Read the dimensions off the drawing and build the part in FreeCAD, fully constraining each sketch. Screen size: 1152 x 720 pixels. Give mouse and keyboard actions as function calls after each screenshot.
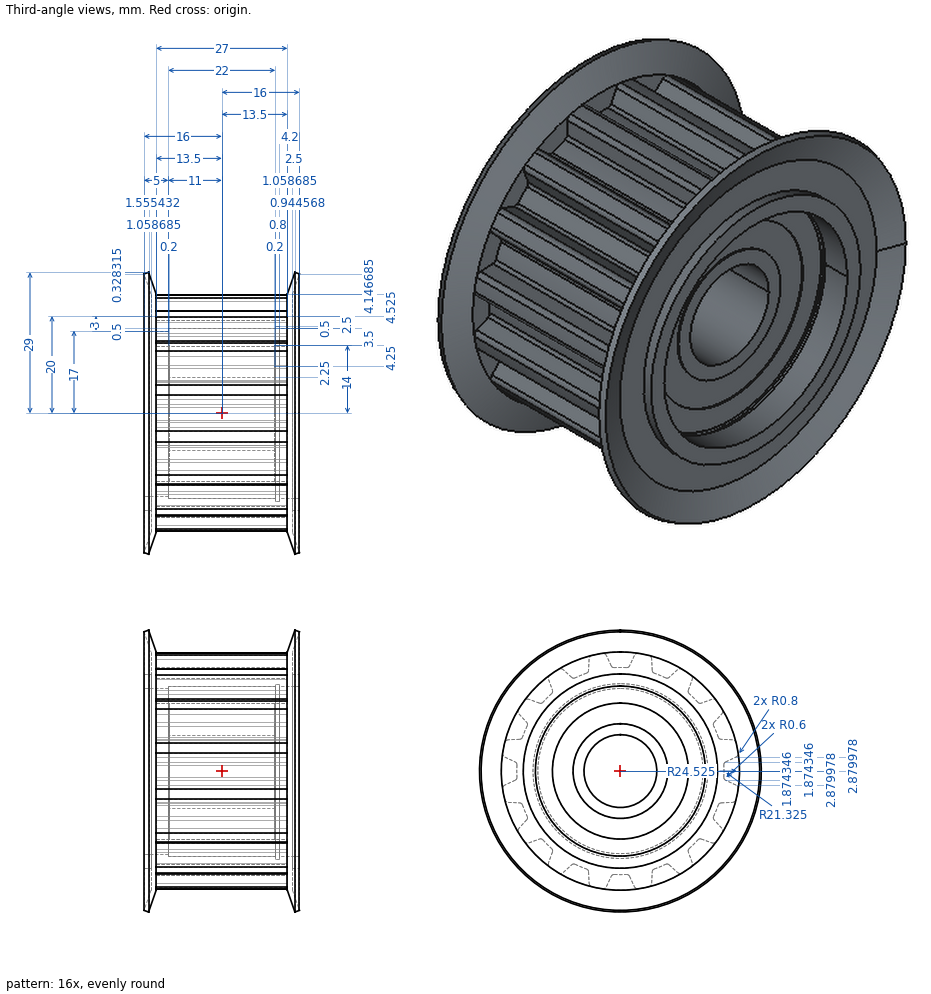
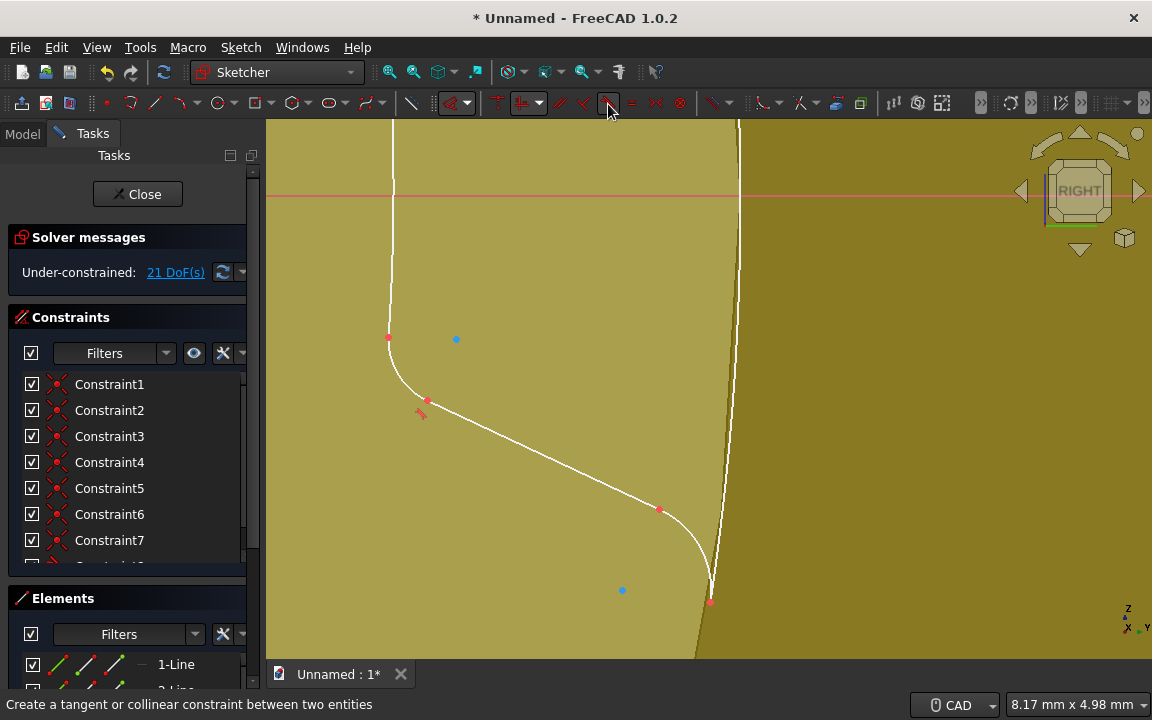
click(590, 477)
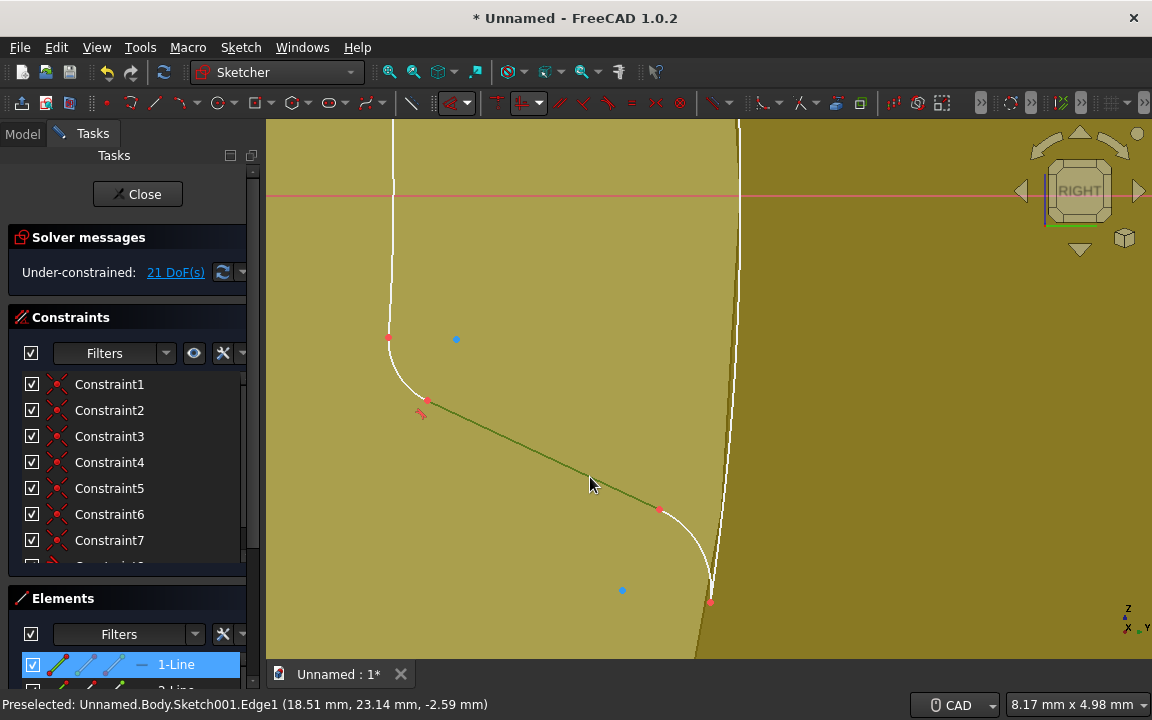
click(687, 530)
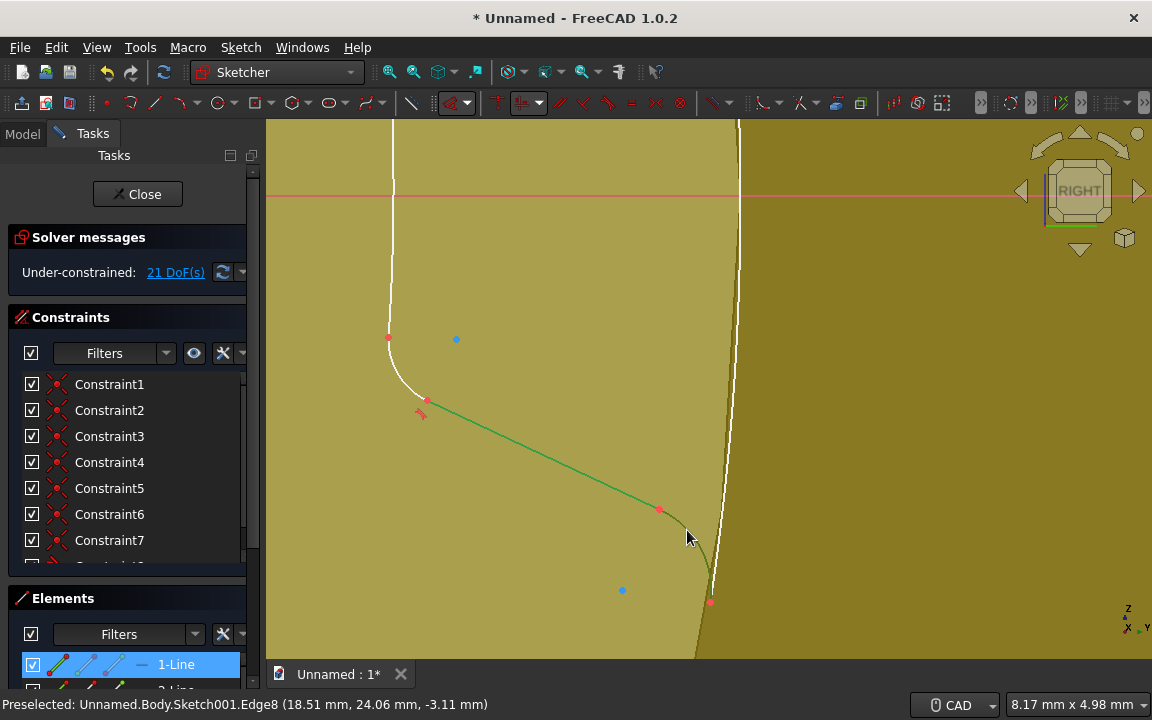
click(608, 104)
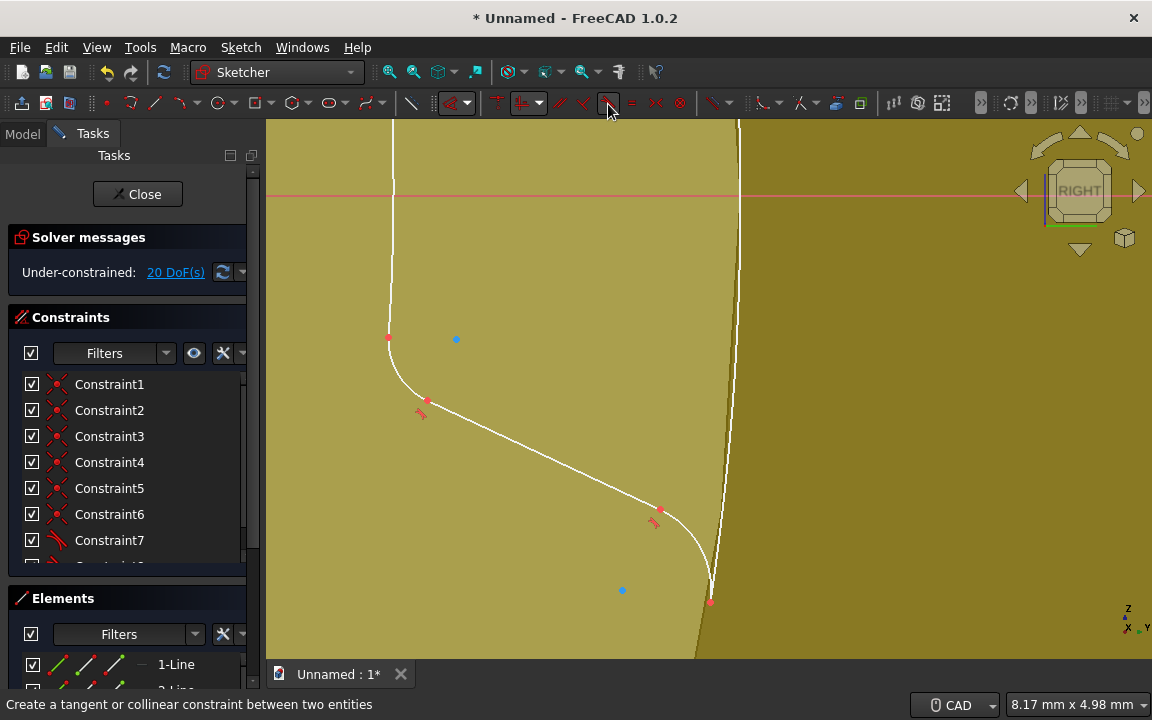
scroll(702, 546, down, 4)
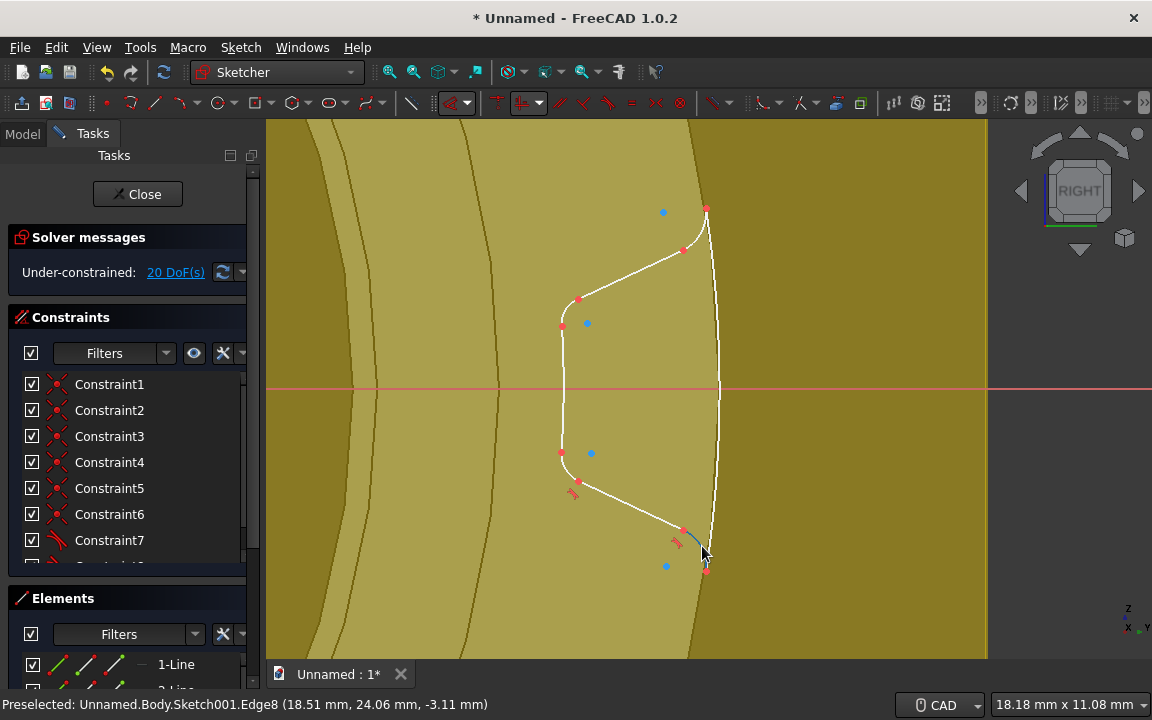
click(610, 285)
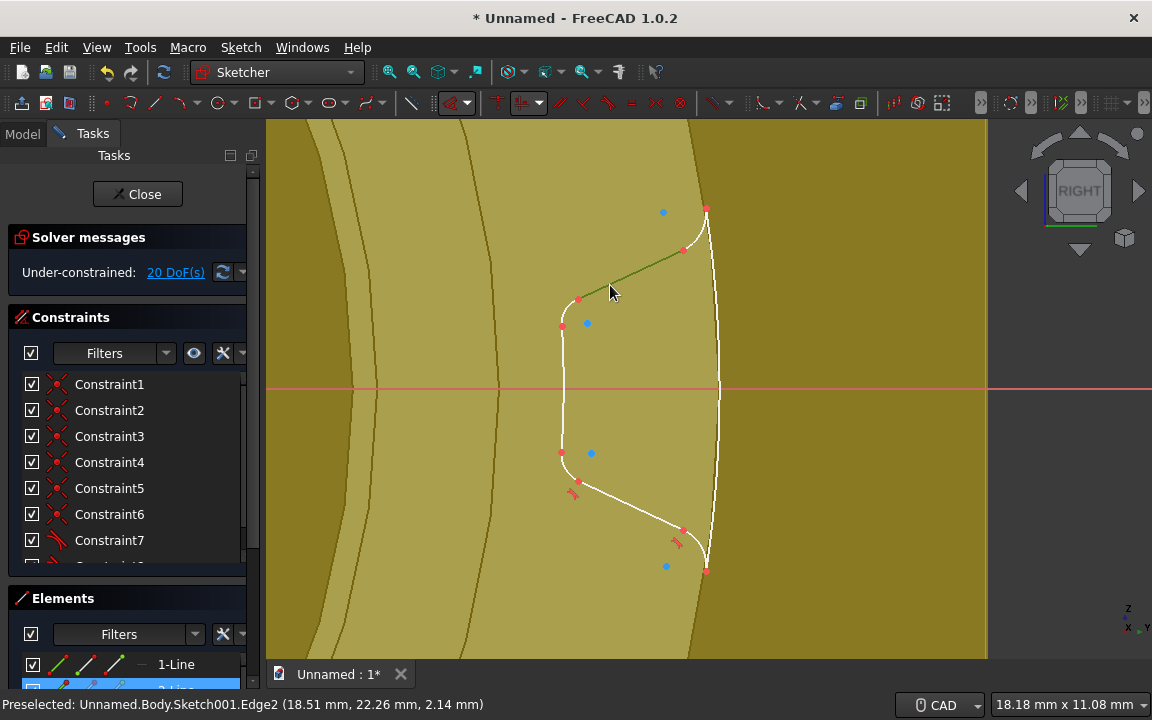
scroll(570, 305, up, 2)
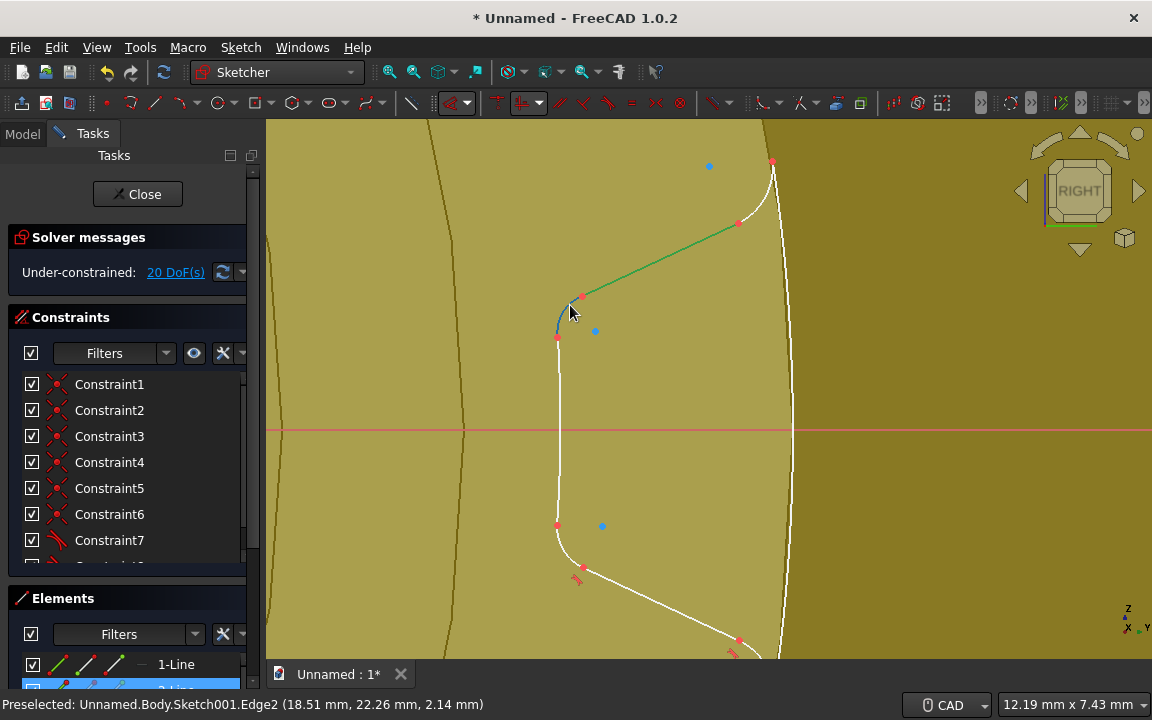
click(569, 304)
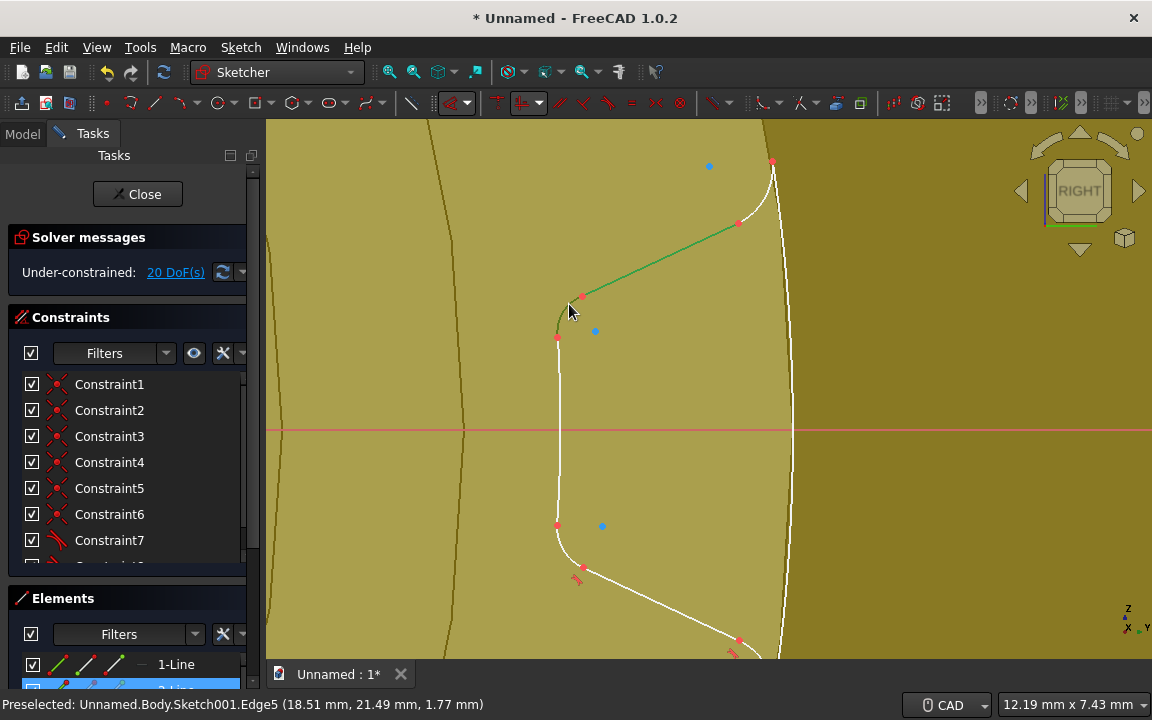
click(608, 104)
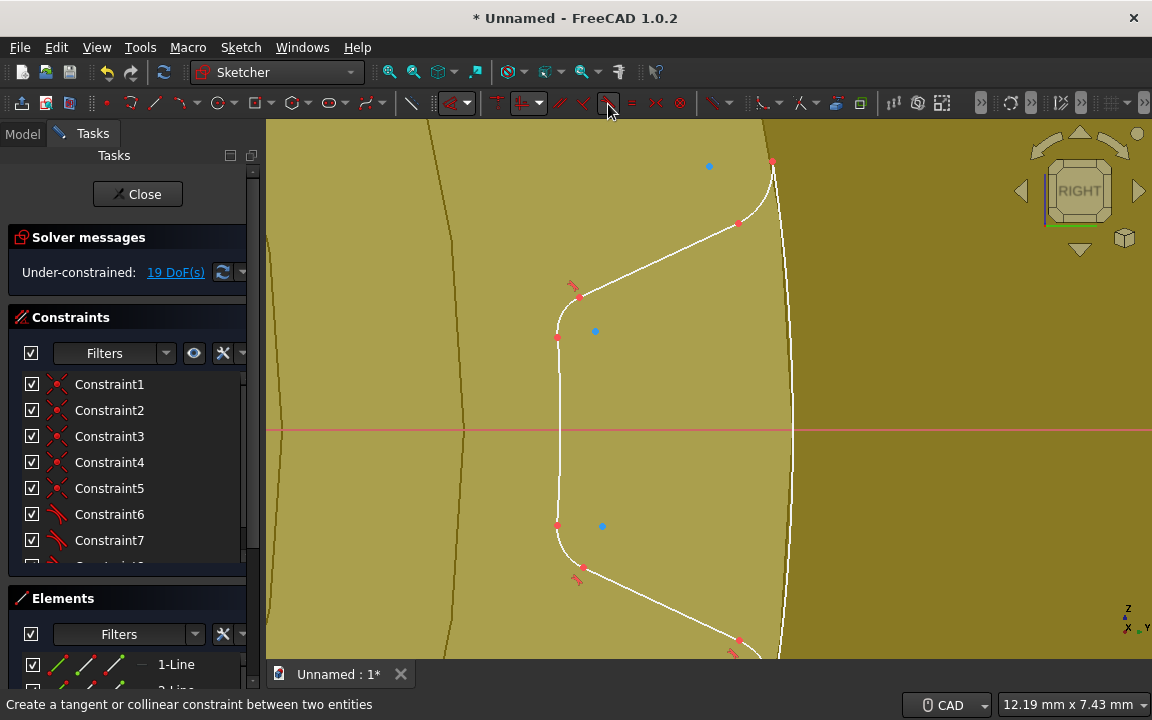
click(627, 275)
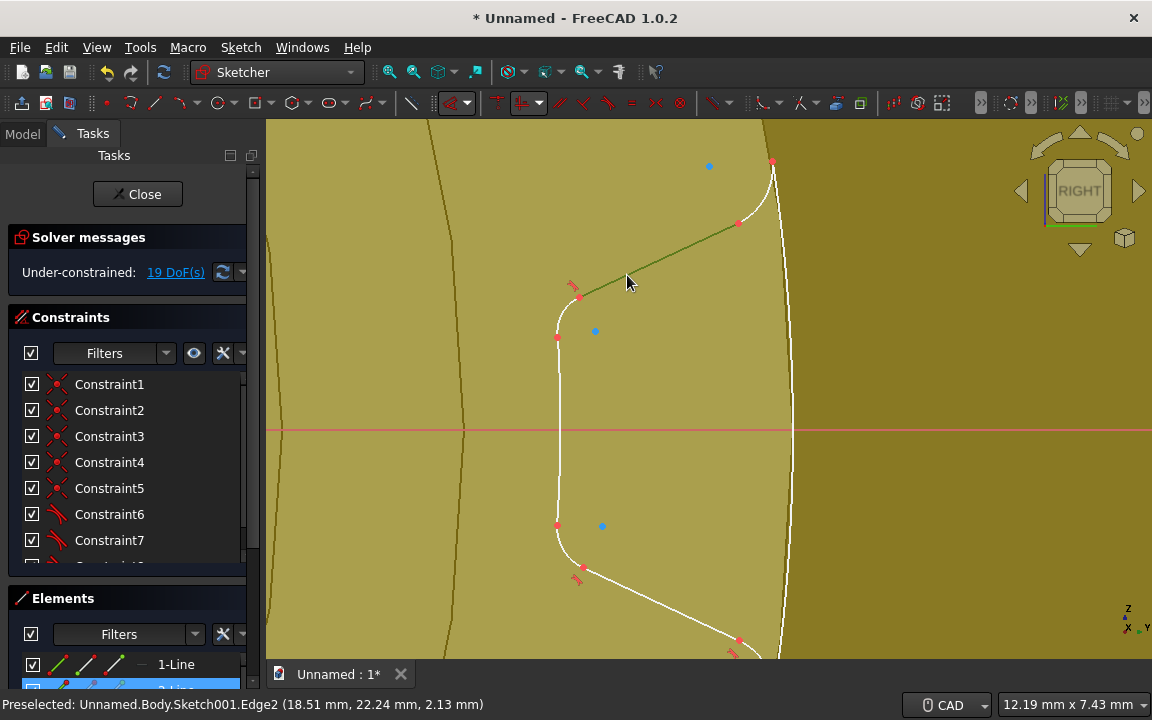
click(757, 209)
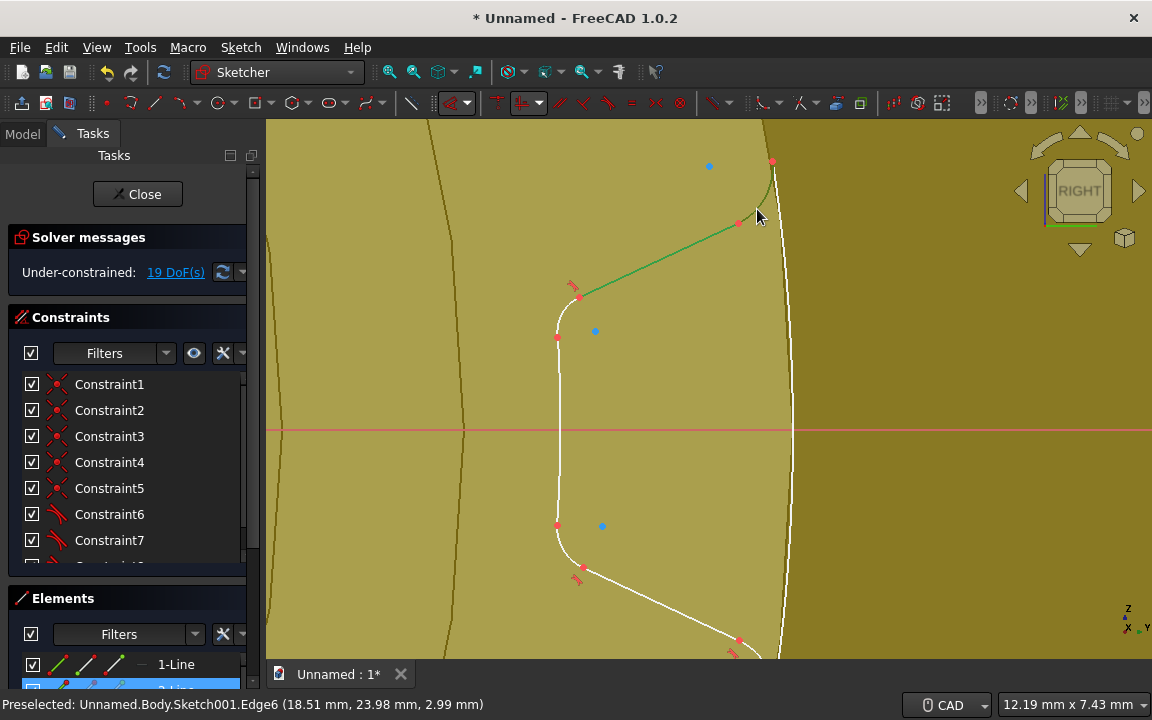
click(608, 104)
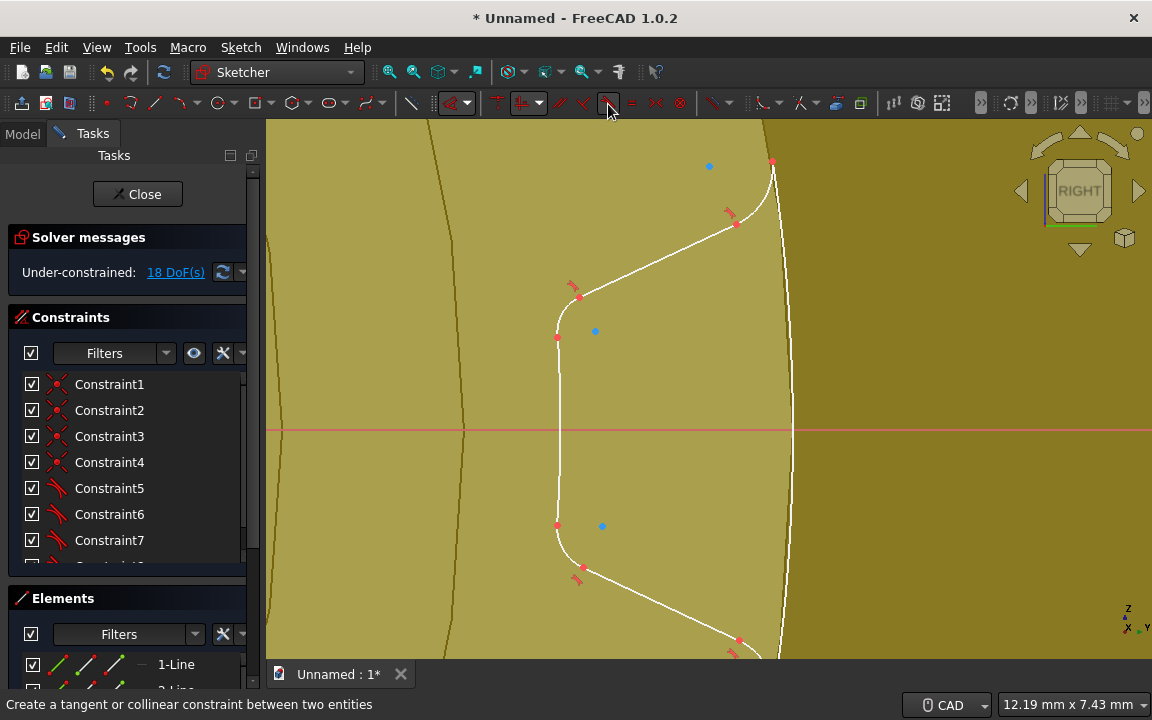
click(559, 541)